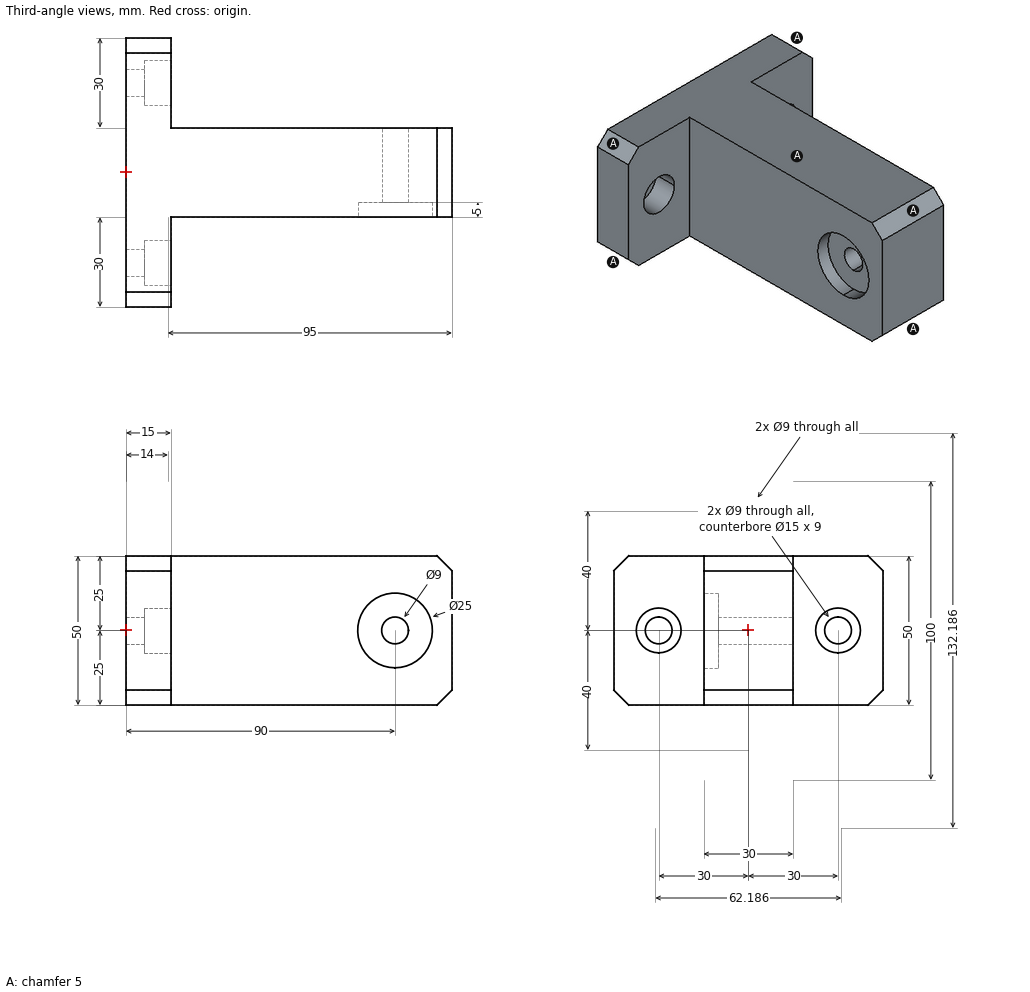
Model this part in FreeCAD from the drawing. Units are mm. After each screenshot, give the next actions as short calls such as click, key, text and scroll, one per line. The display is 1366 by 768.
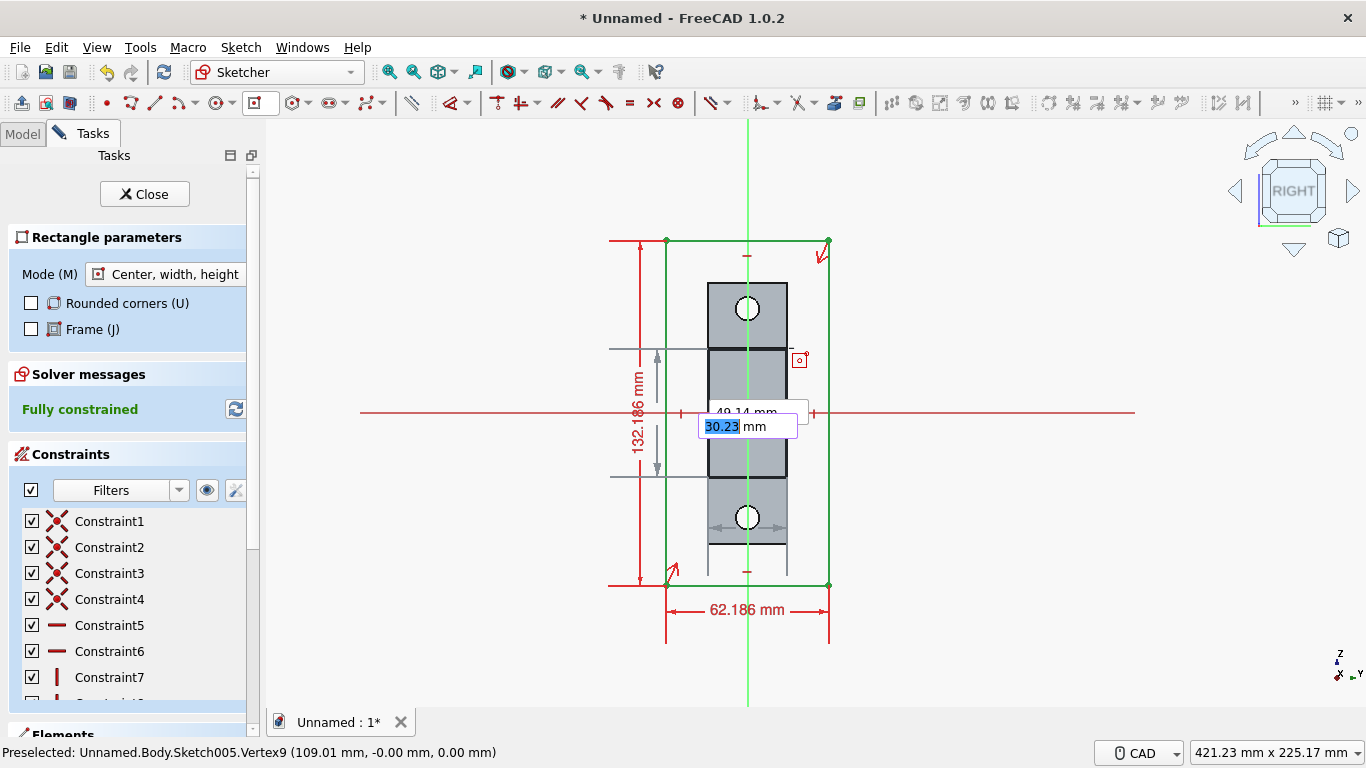
text(30)
key(Tab)
text(50)
key(Return)
key(Escape)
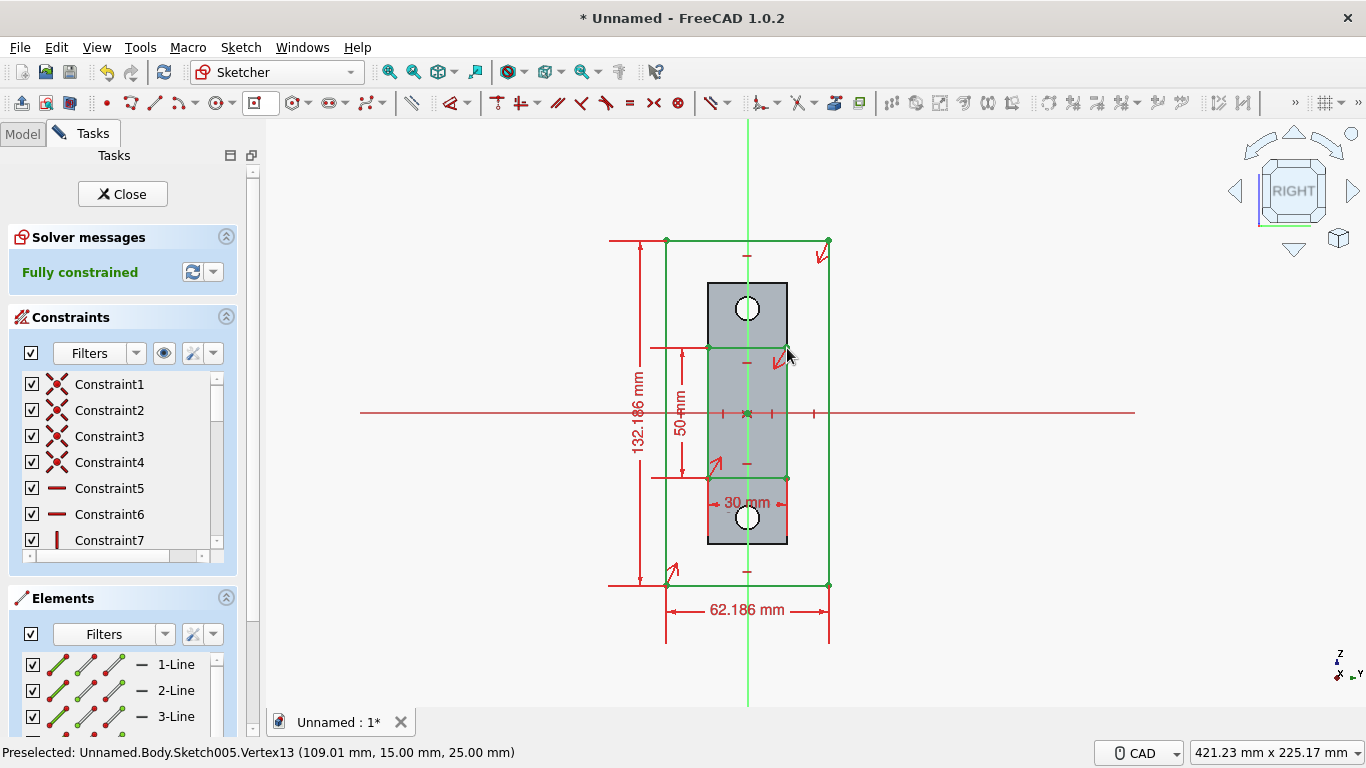
click(123, 194)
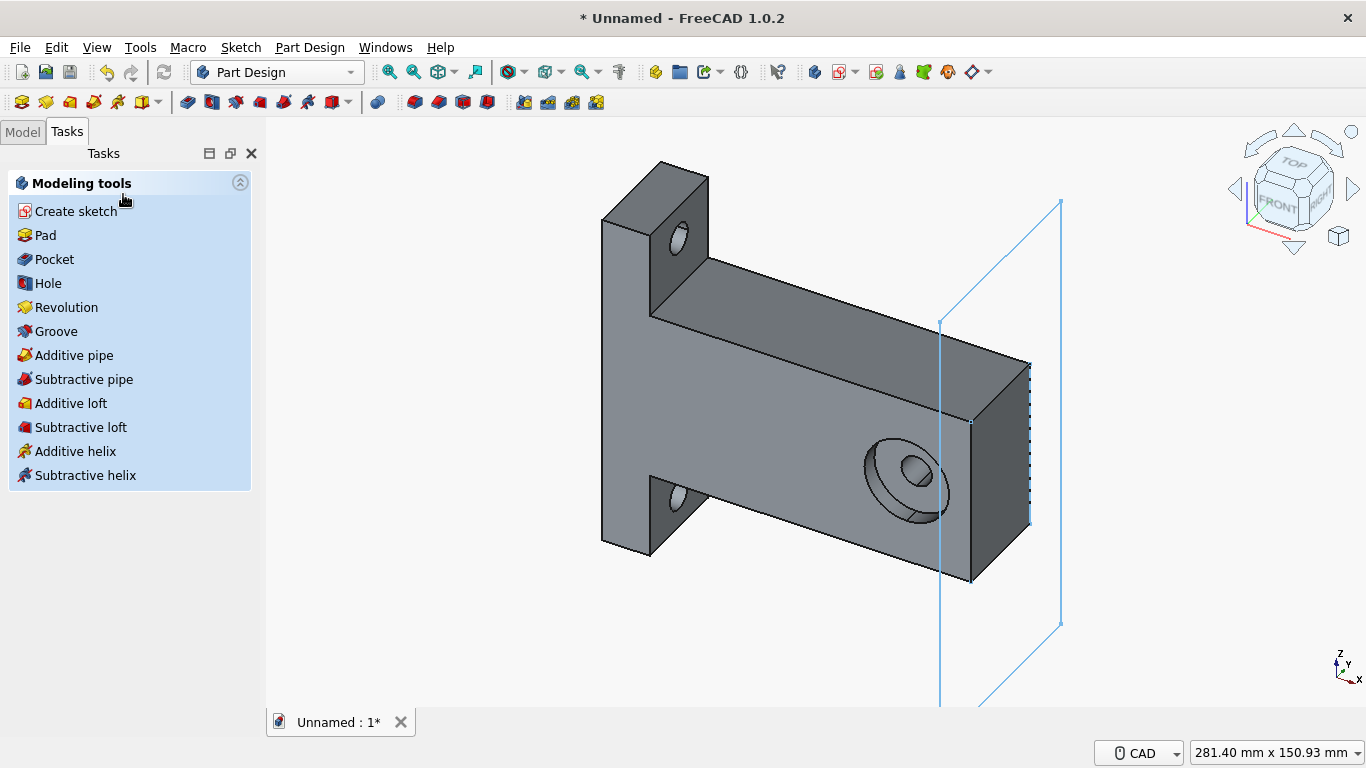
click(188, 102)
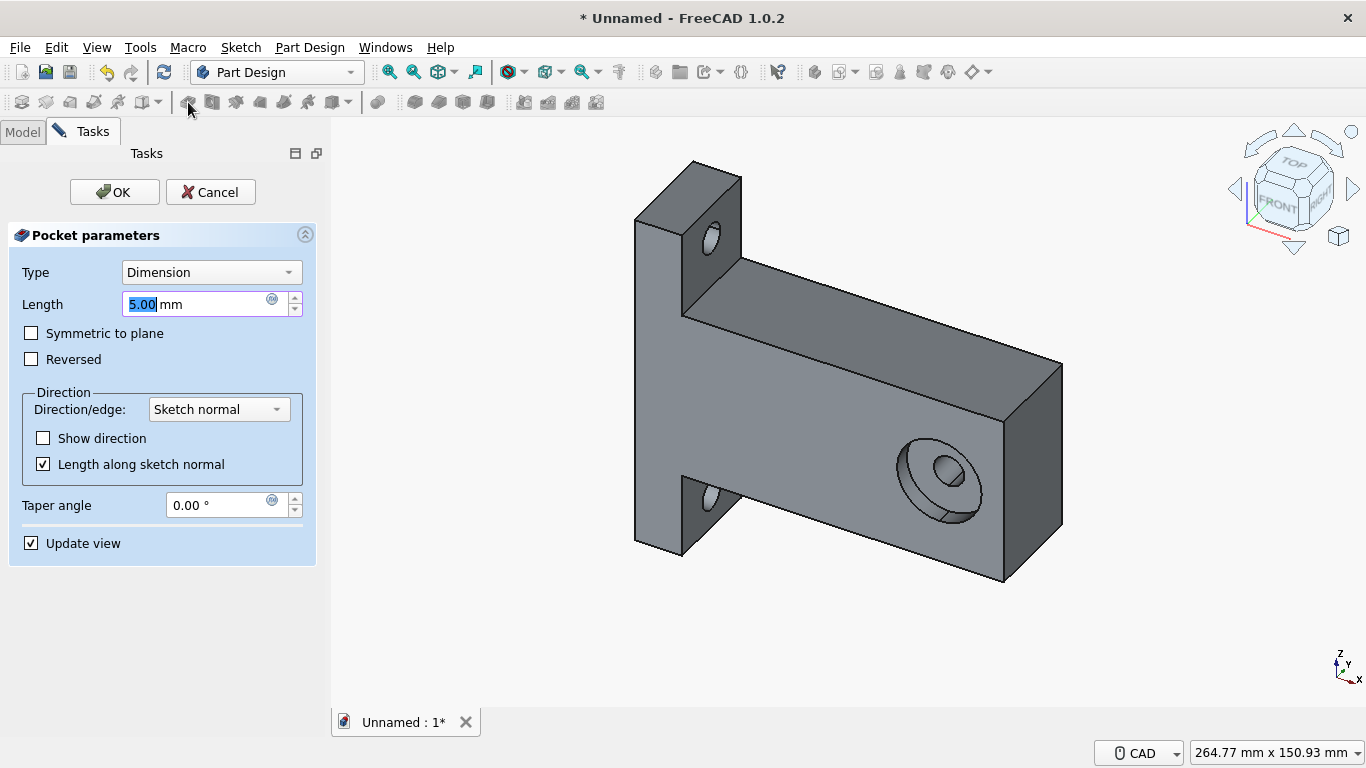
click(212, 272)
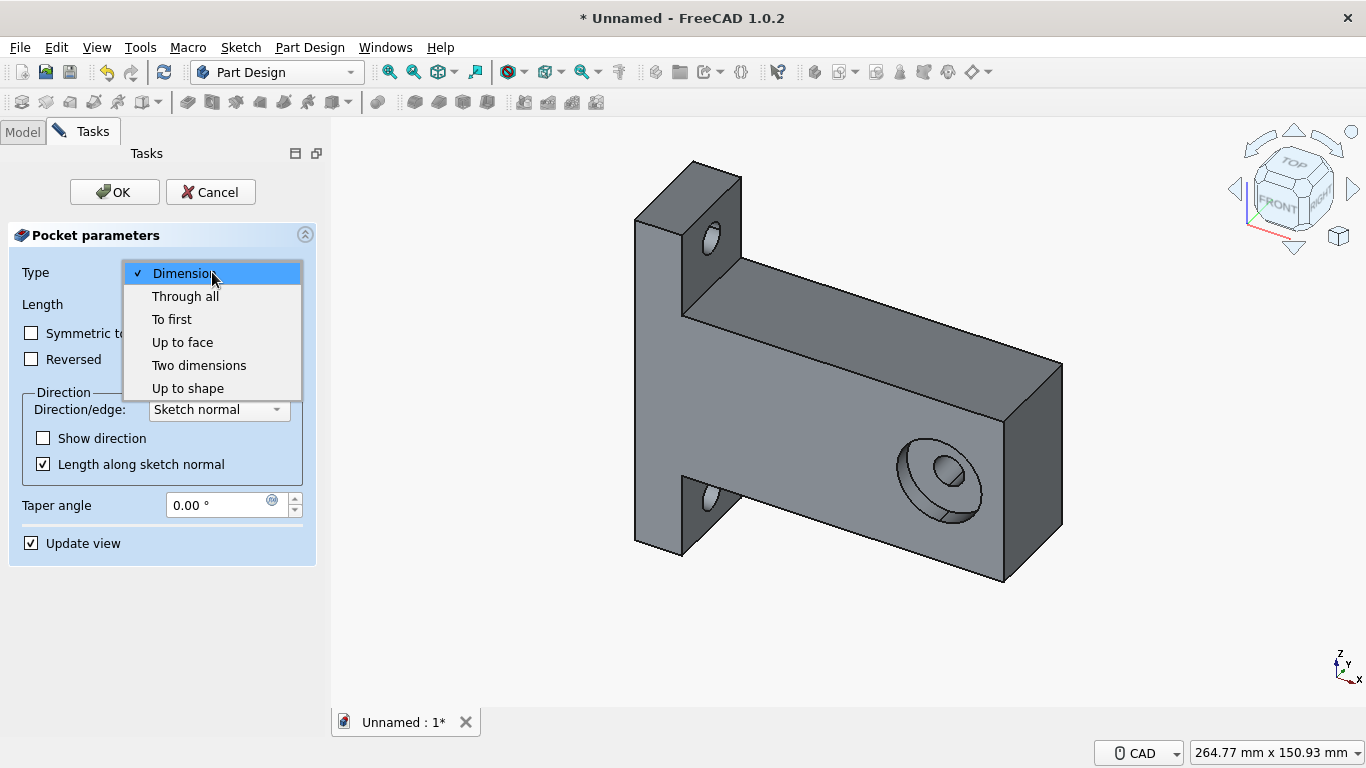
click(212, 296)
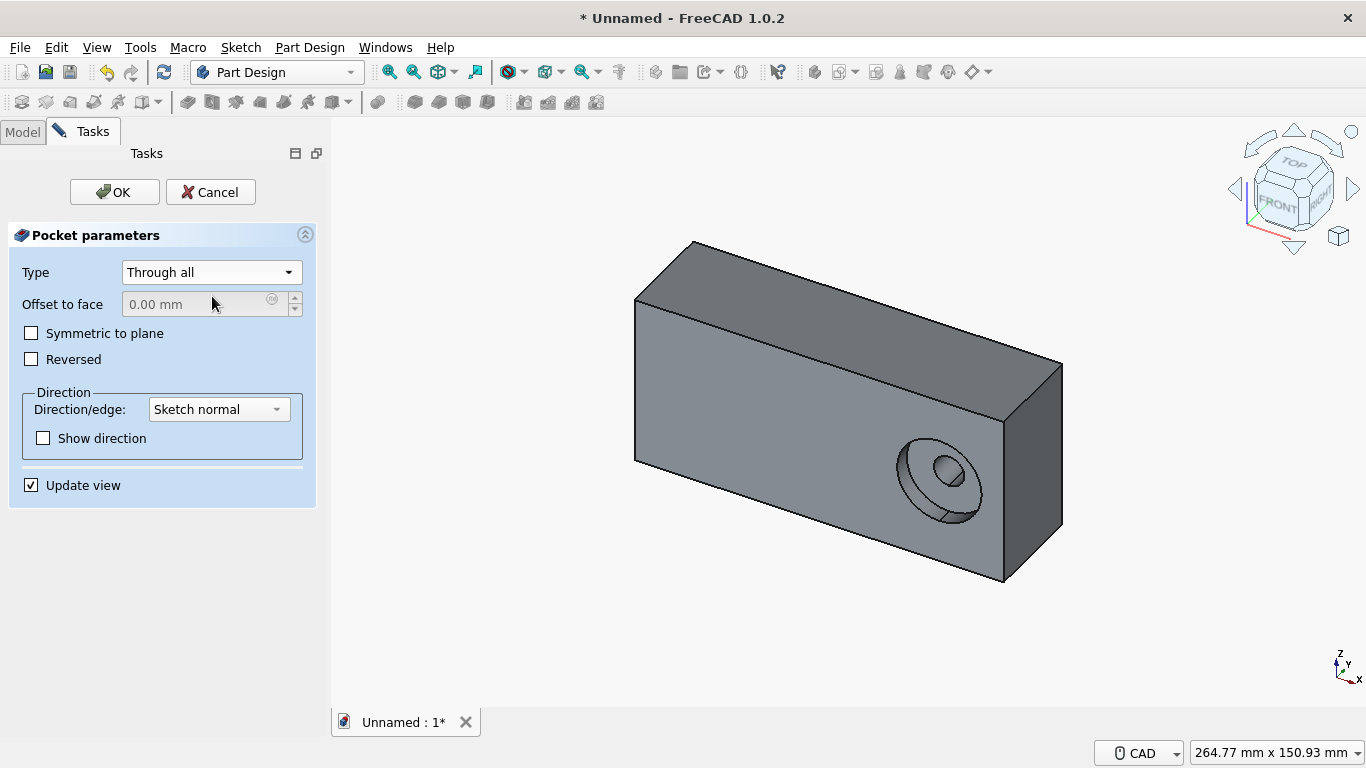
click(115, 192)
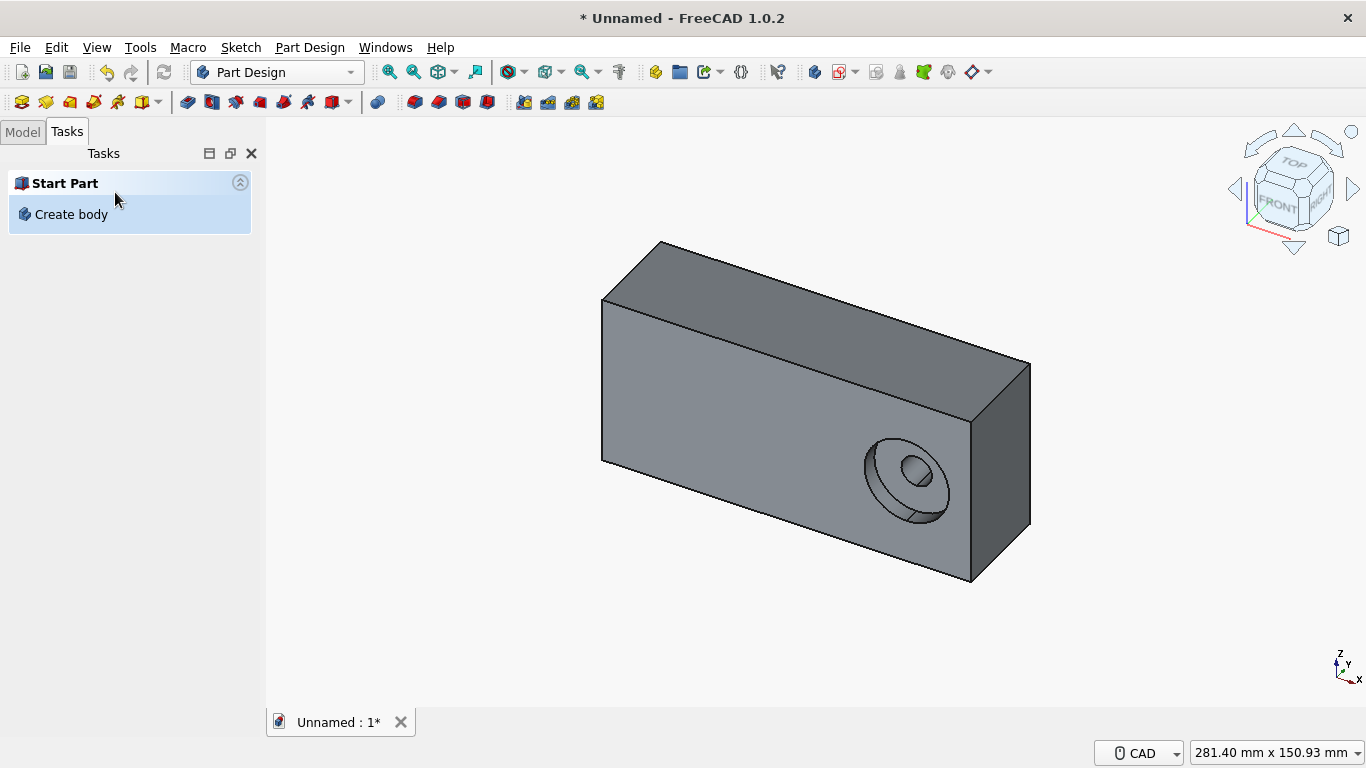
click(734, 423)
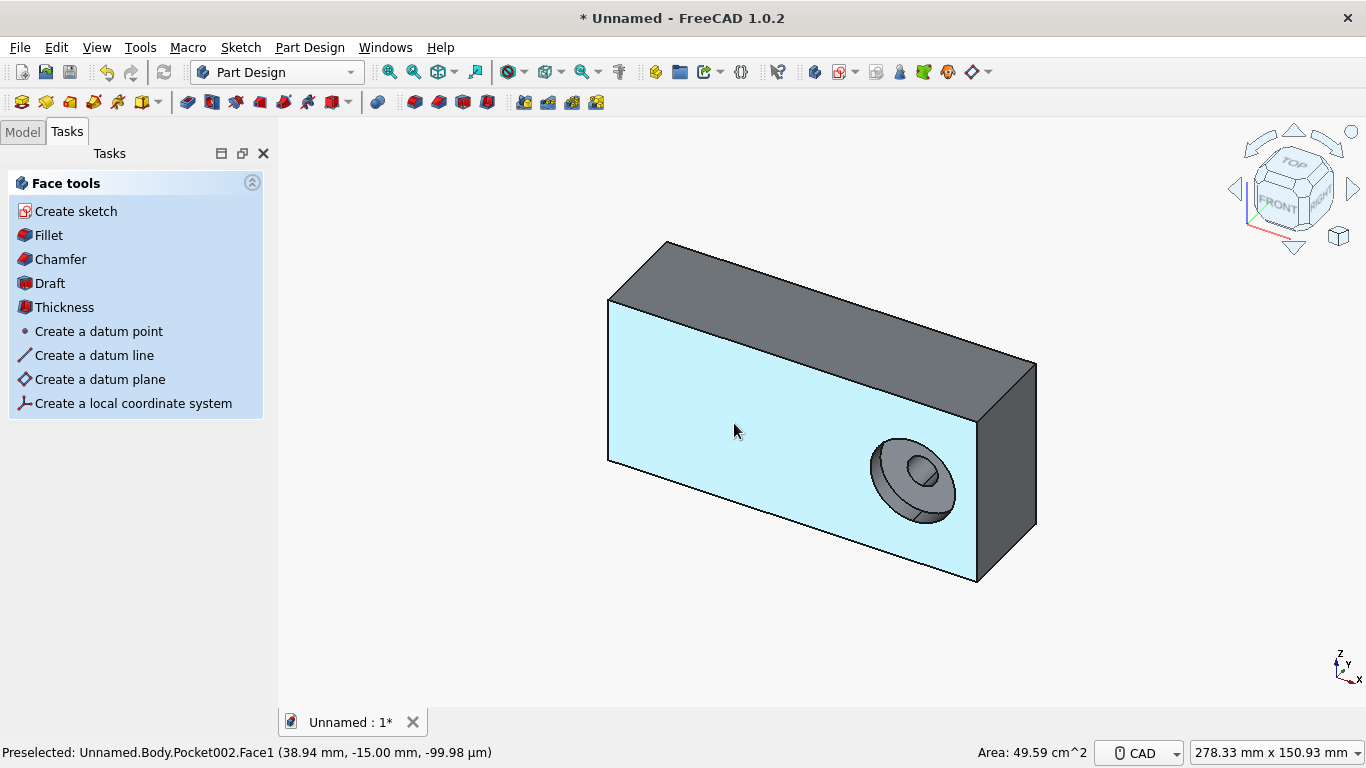
click(840, 72)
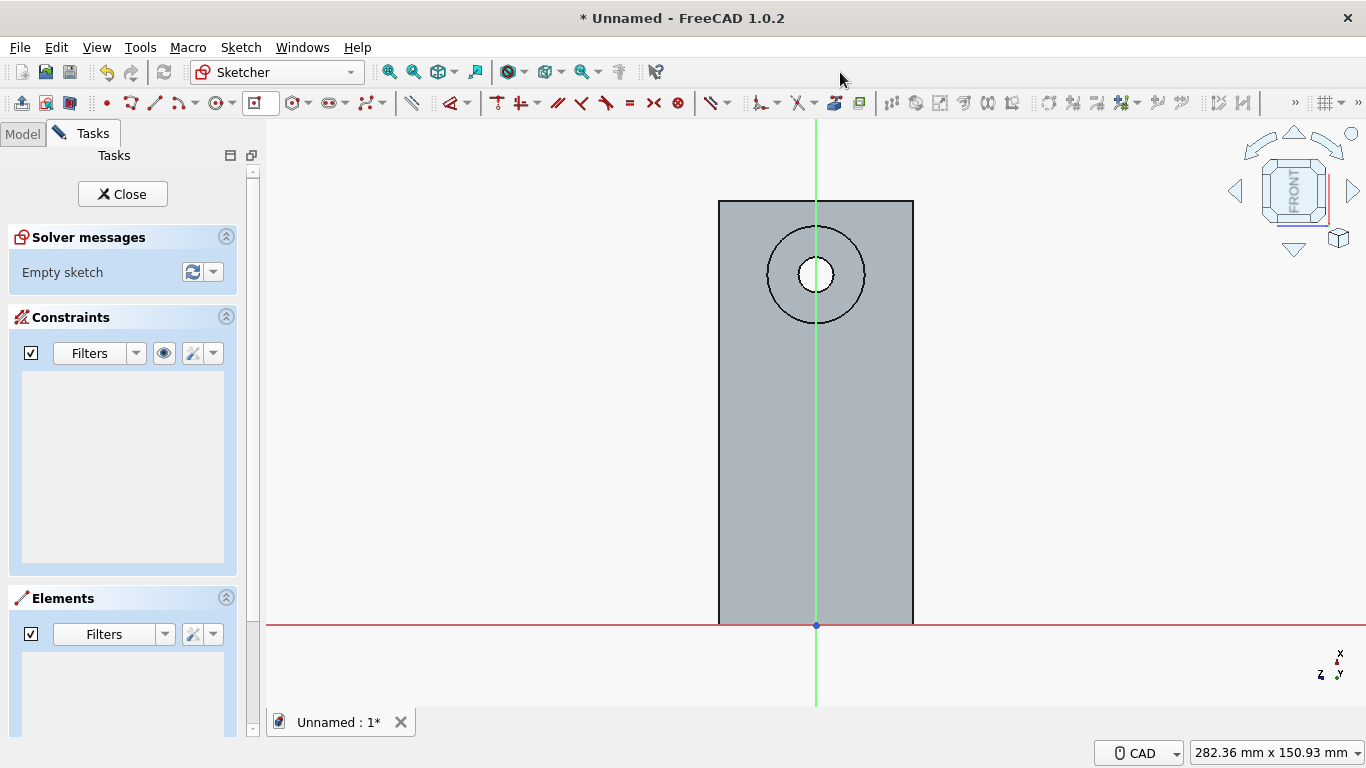
scroll(846, 675, up, 6)